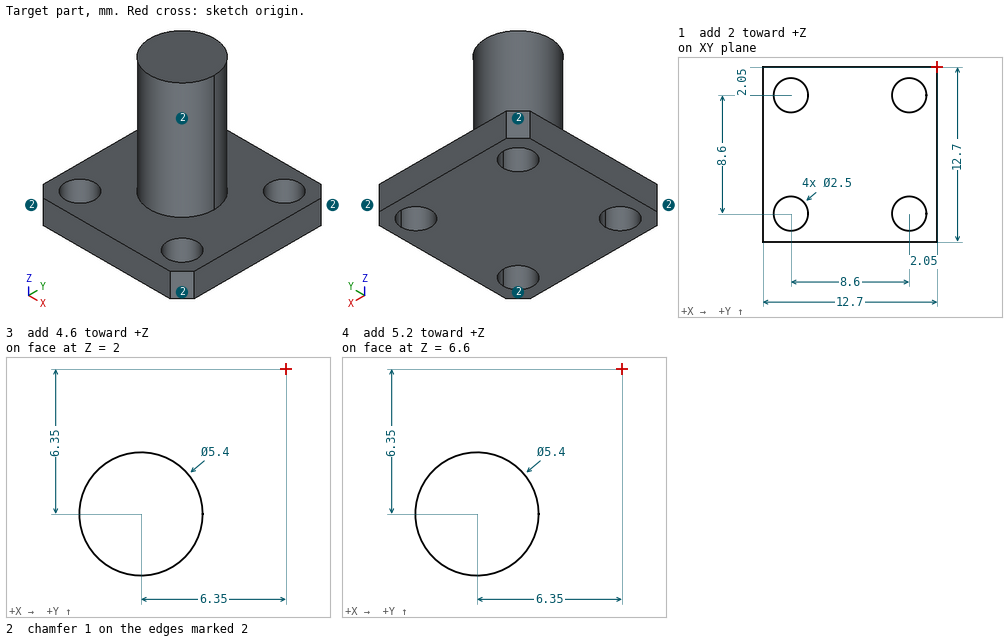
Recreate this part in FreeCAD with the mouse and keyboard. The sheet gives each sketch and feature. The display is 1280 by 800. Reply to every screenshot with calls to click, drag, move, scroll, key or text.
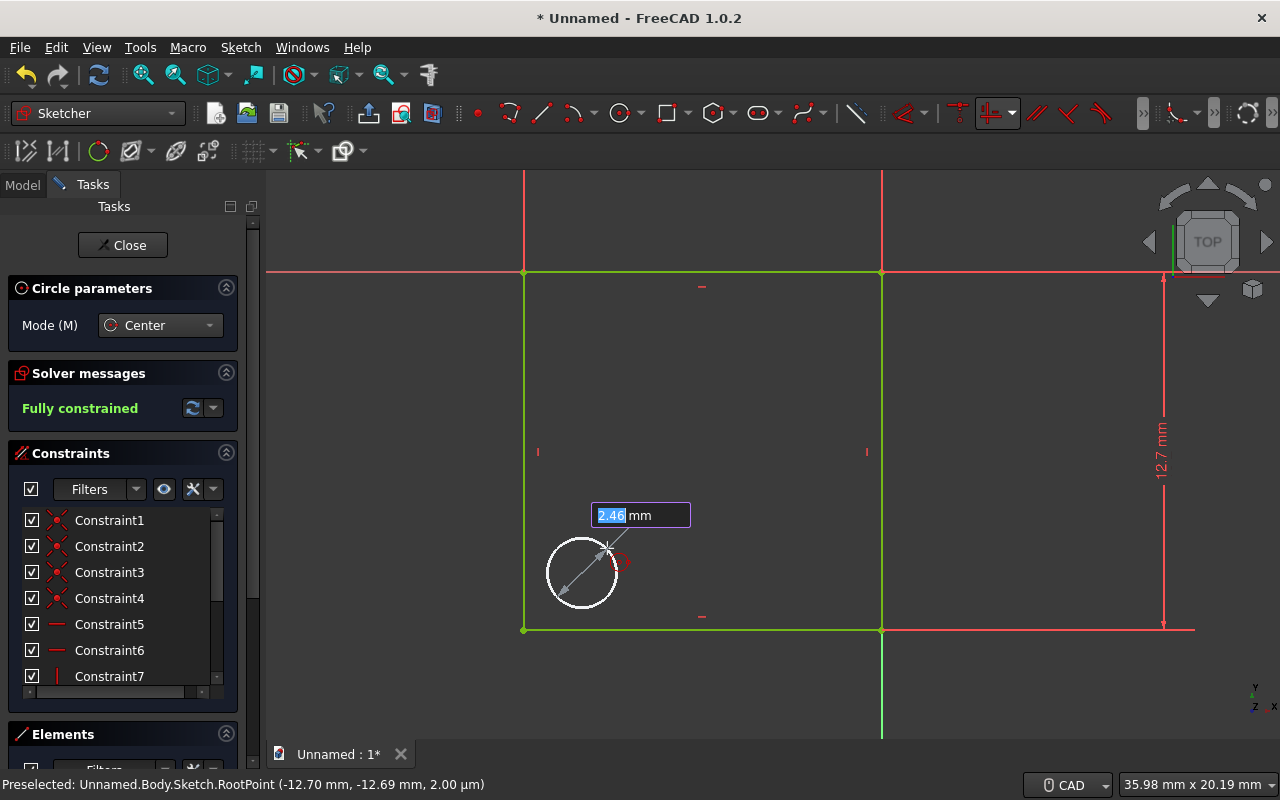
text(2.5)
key(Return)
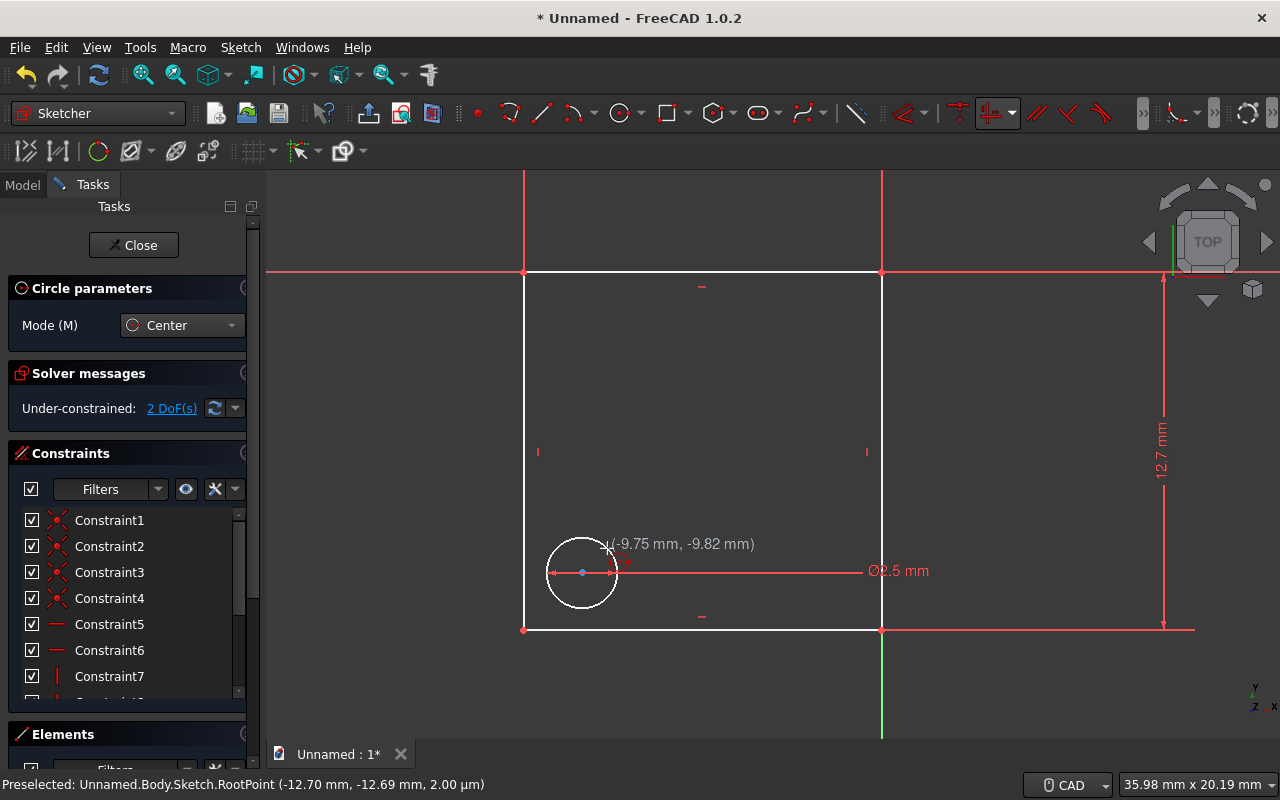
click(824, 572)
move(849, 548)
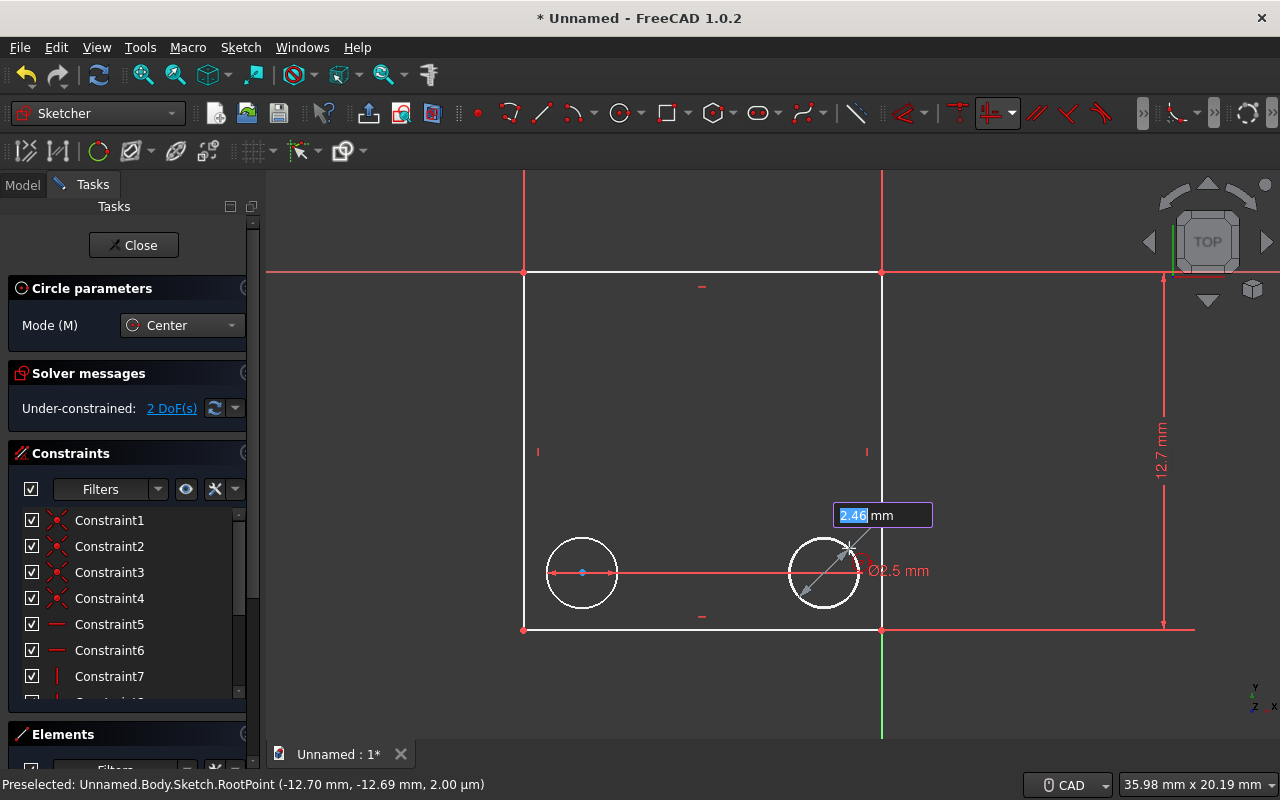
text(2.5)
key(Return)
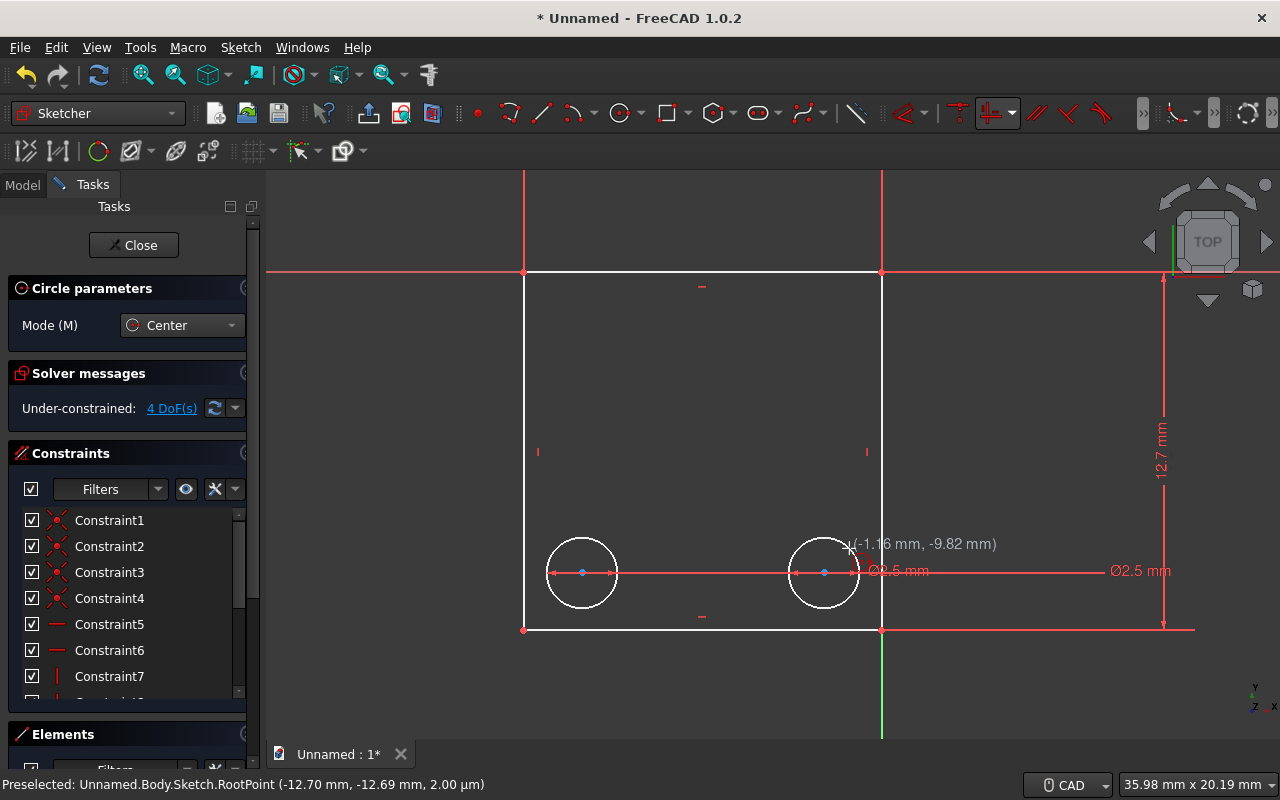
click(582, 330)
move(607, 305)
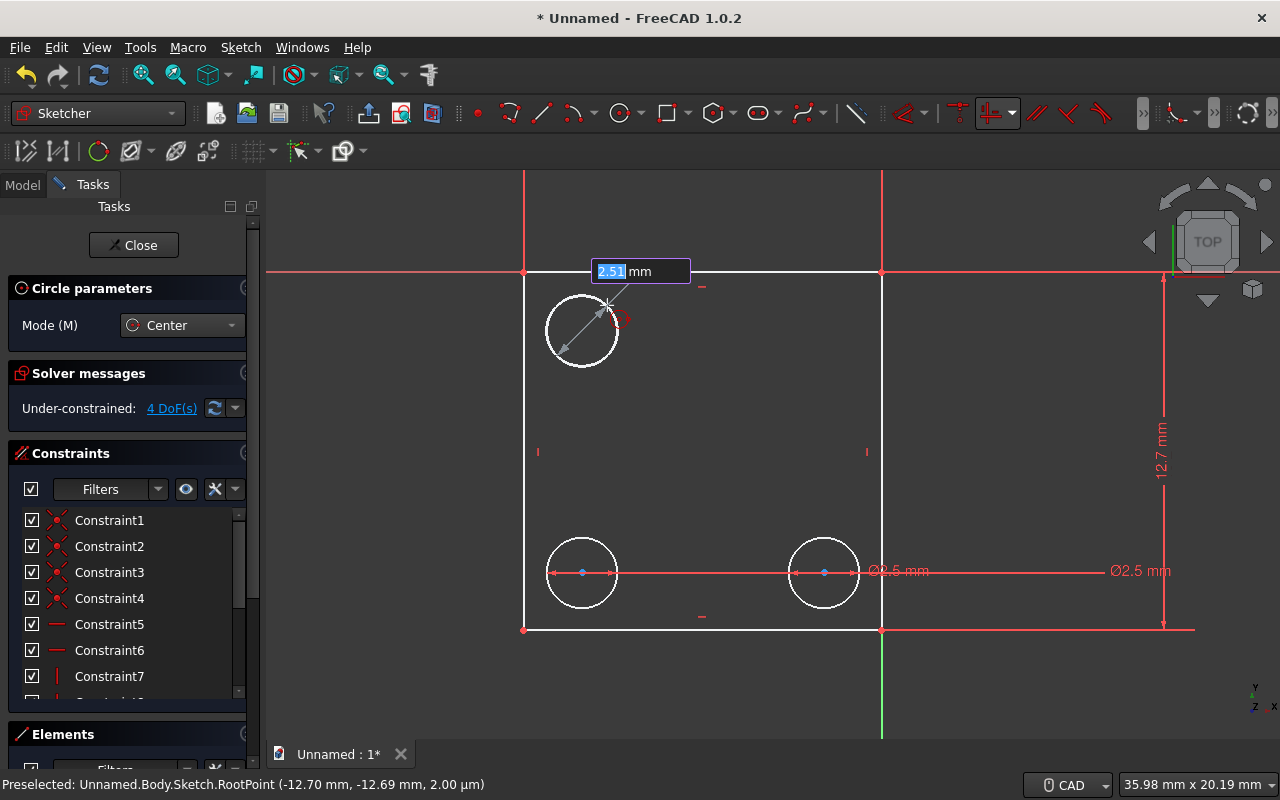
text(2.5)
key(Return)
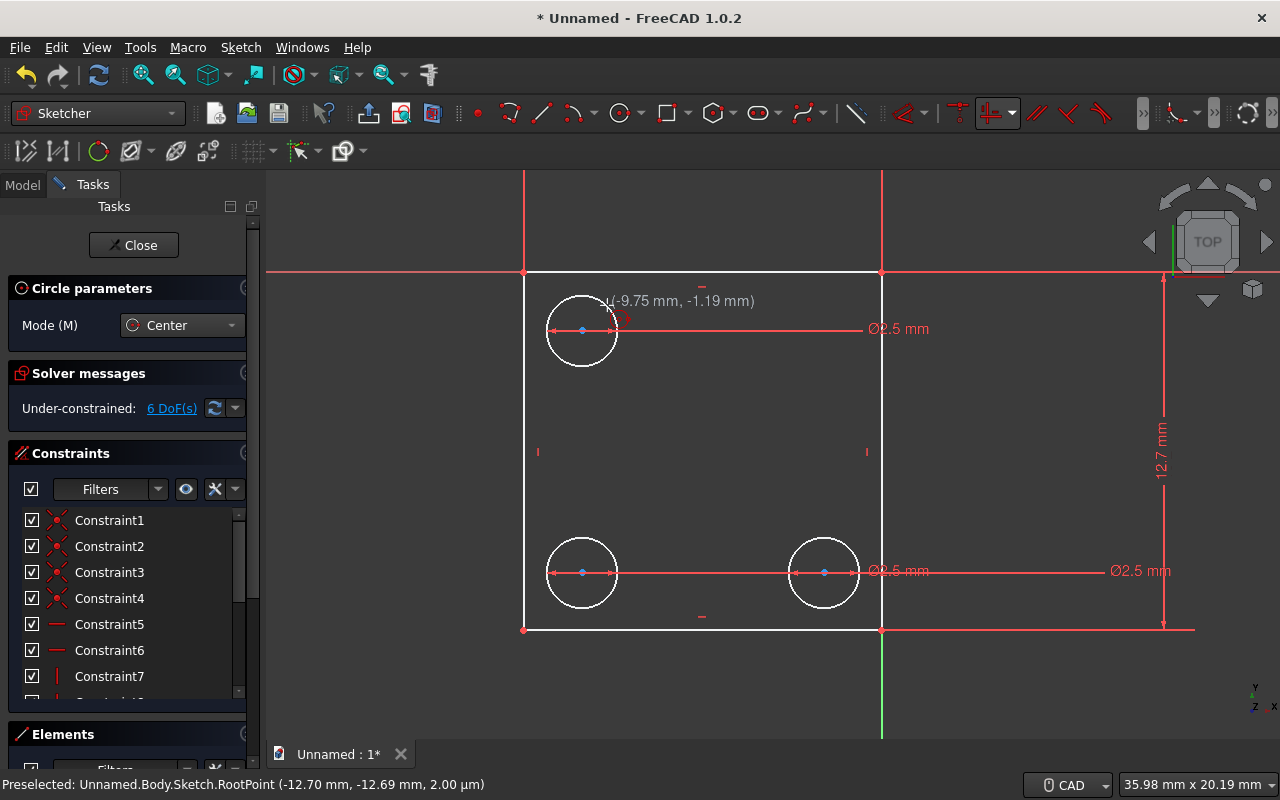
click(824, 330)
move(849, 305)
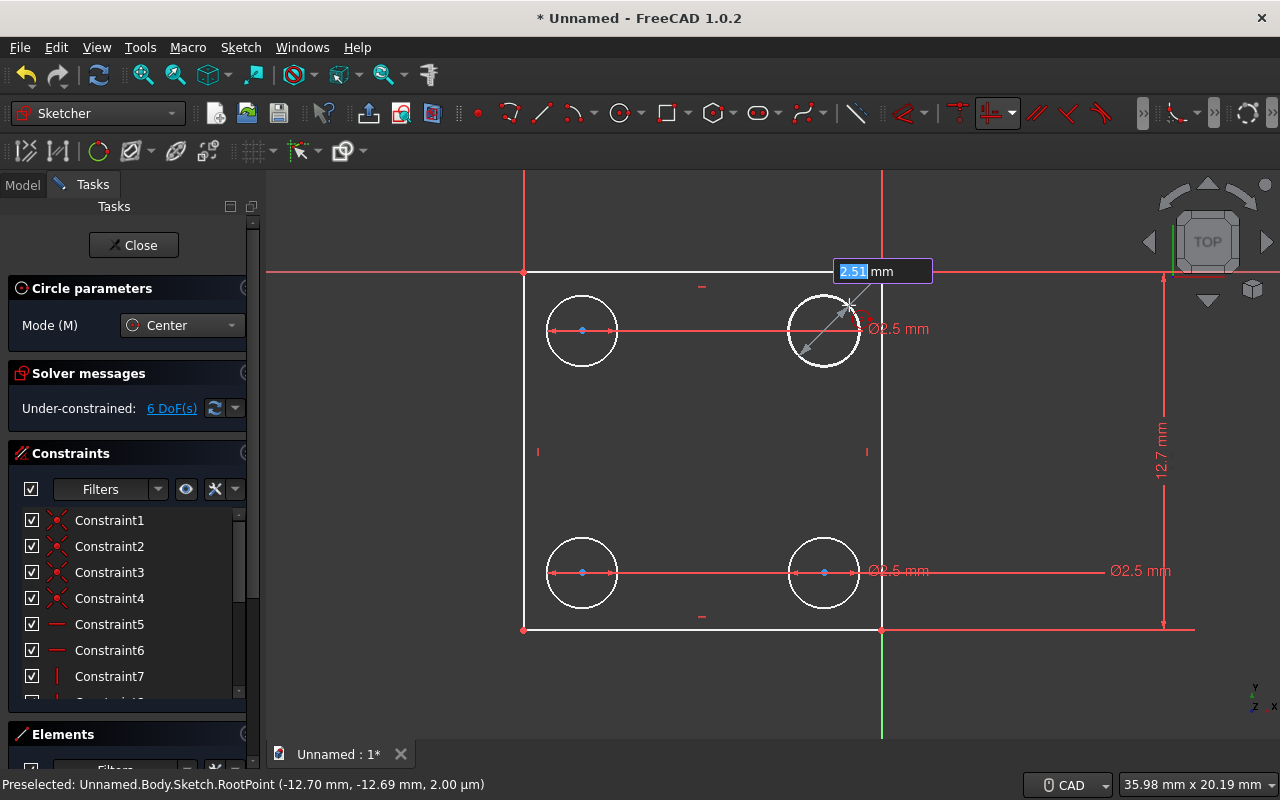
text(2.5)
key(Return)
key(Escape)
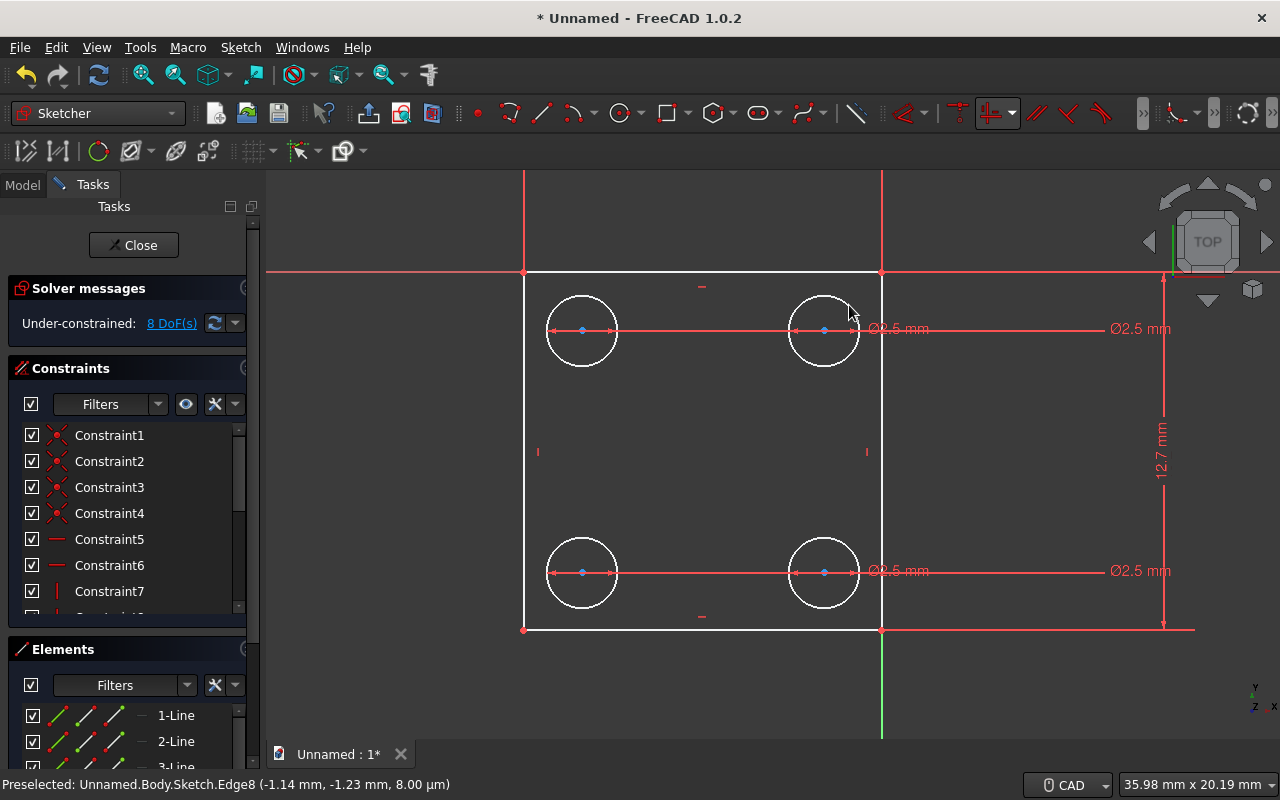
click(582, 573)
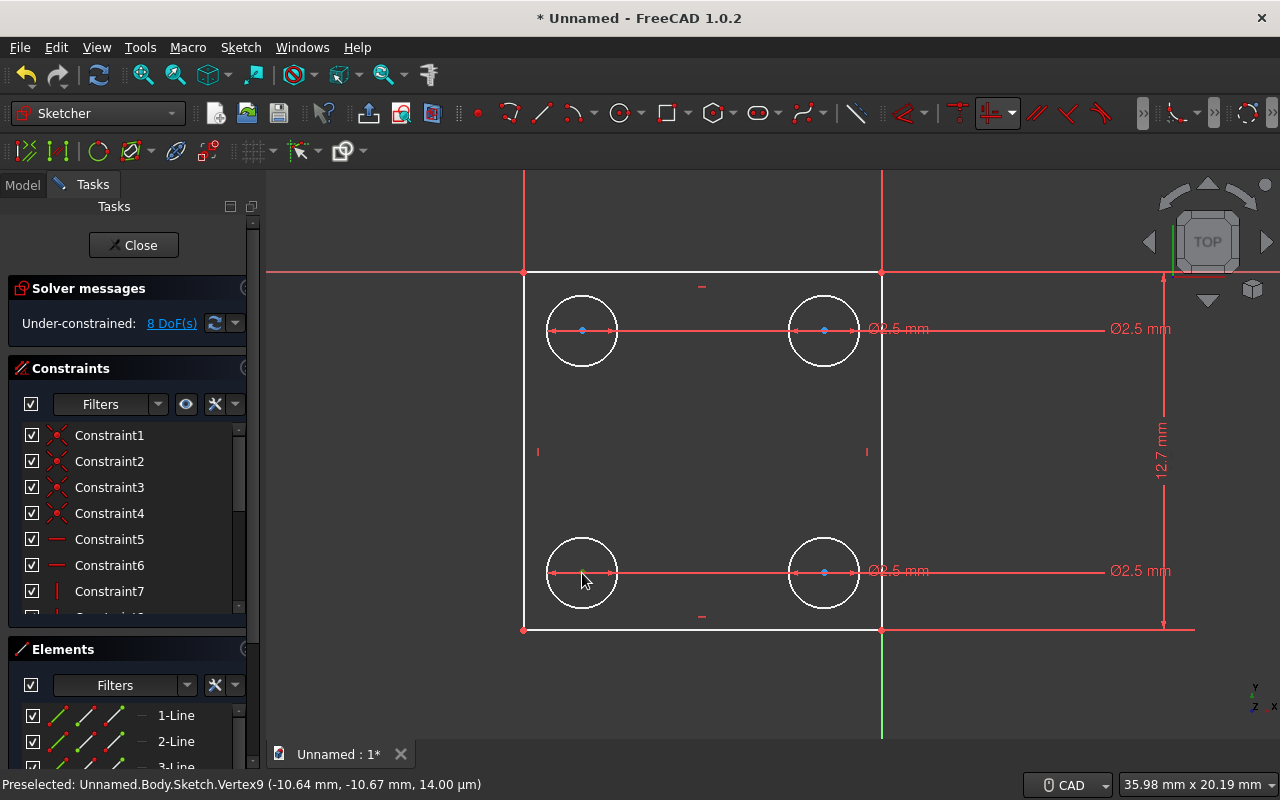
click(824, 573)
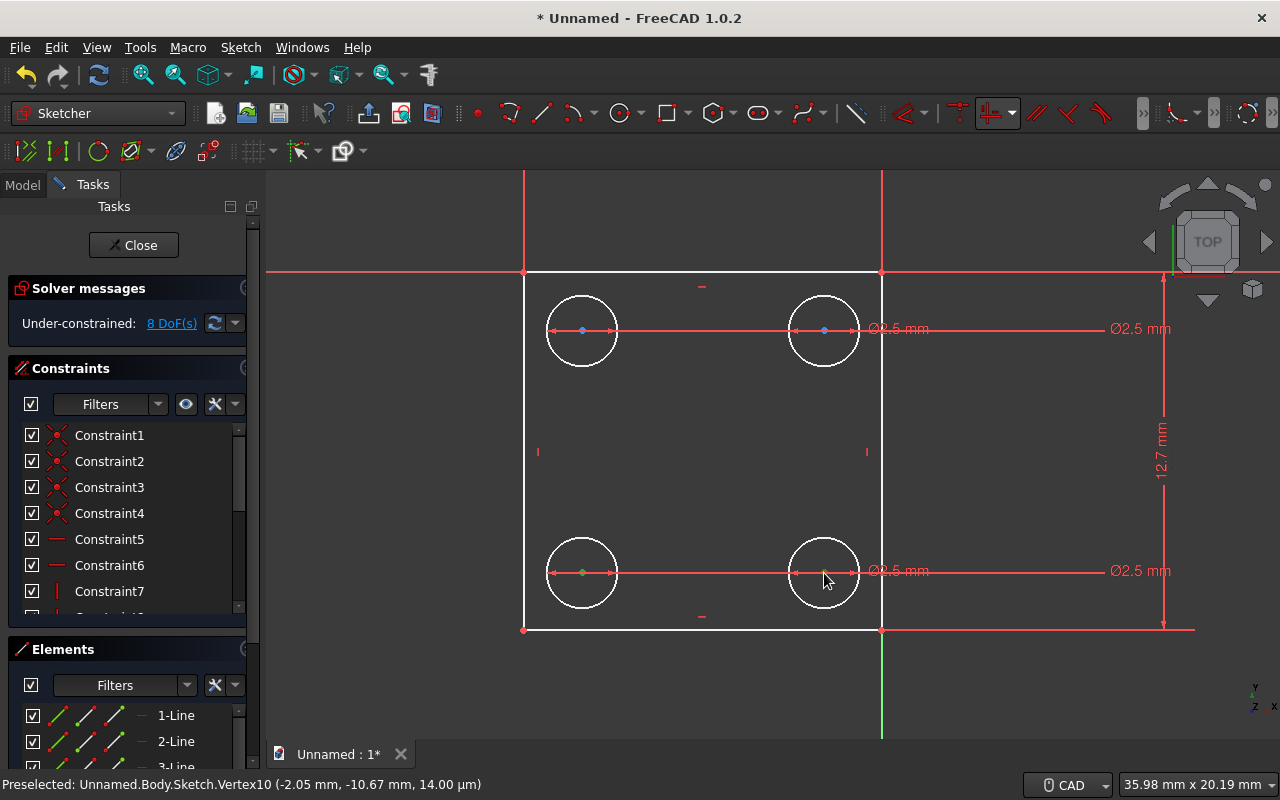
click(1014, 114)